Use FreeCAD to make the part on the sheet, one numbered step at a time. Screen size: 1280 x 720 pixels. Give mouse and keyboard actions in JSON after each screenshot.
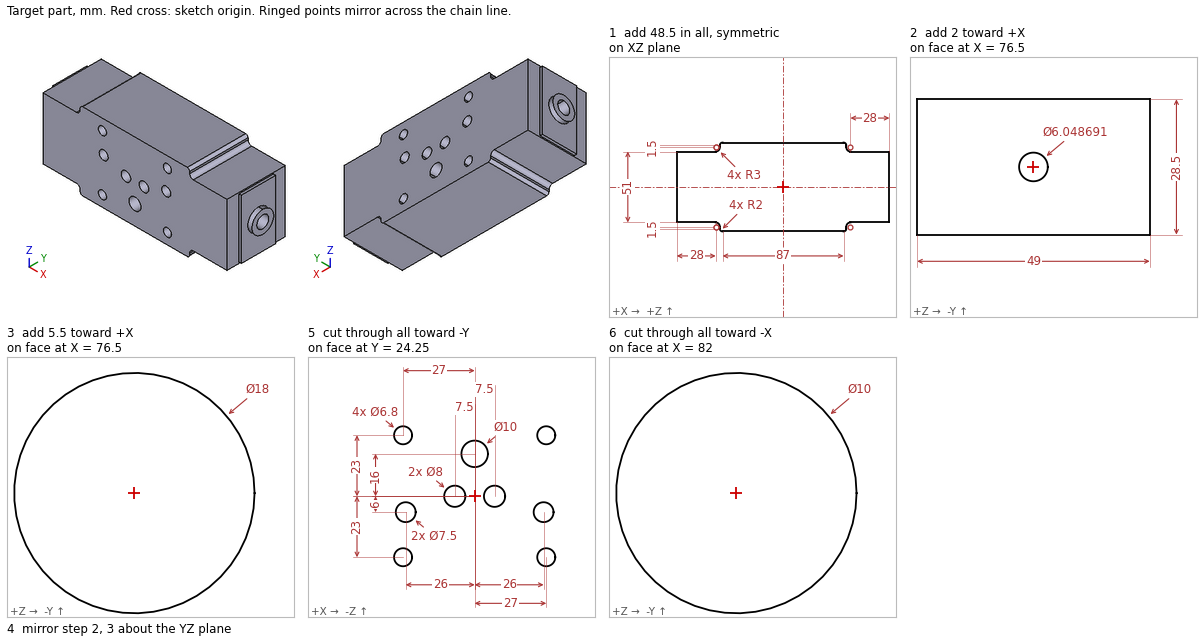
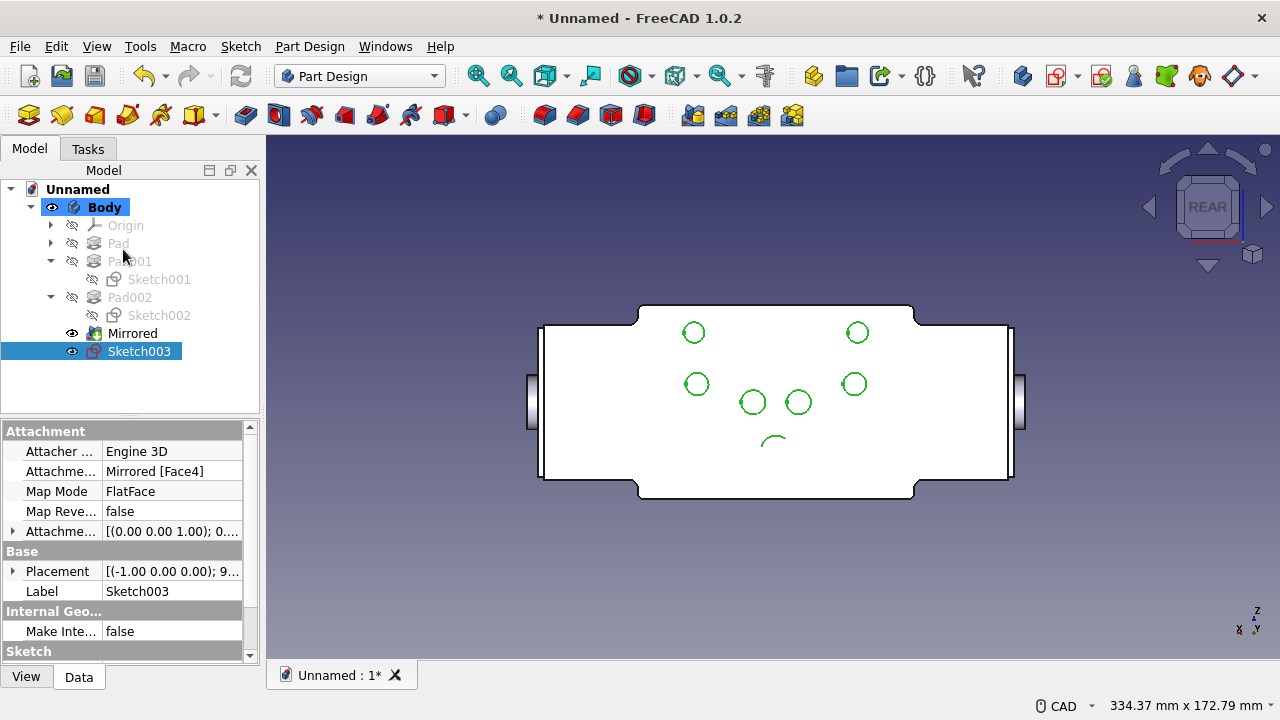
{"action": "left_click", "coordinate": [246, 116]}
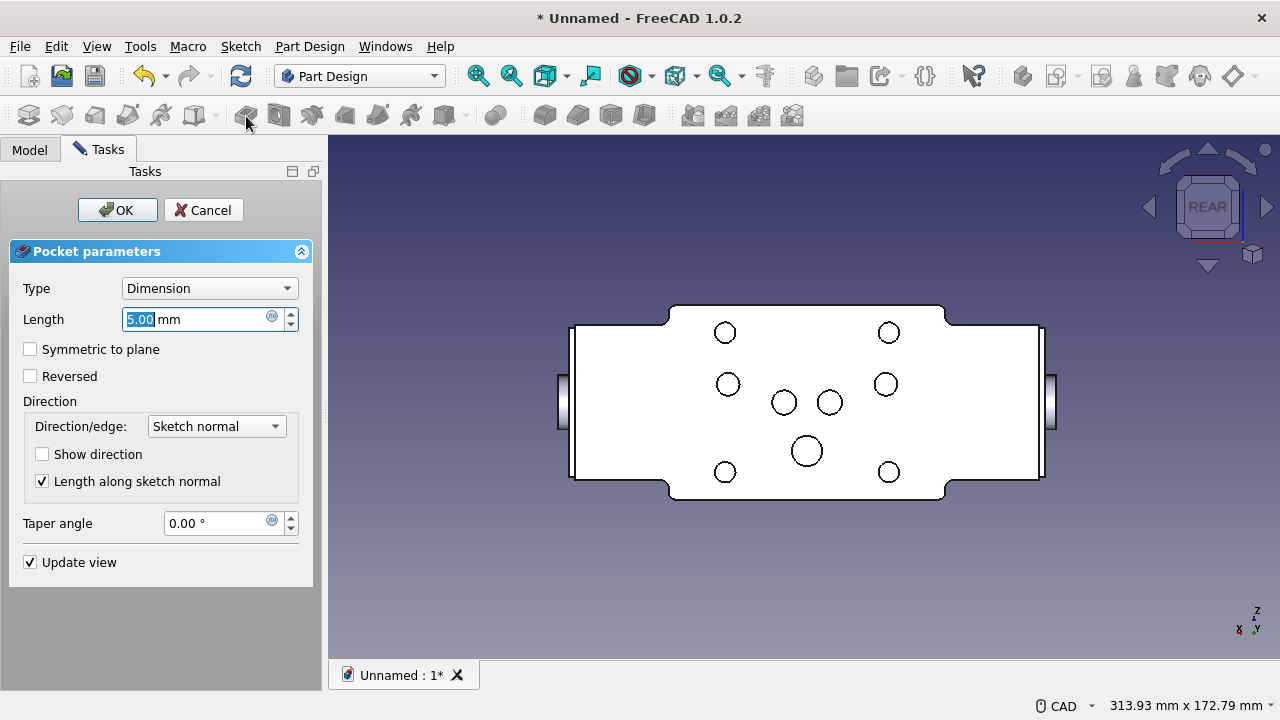
{"action": "left_click", "coordinate": [210, 288]}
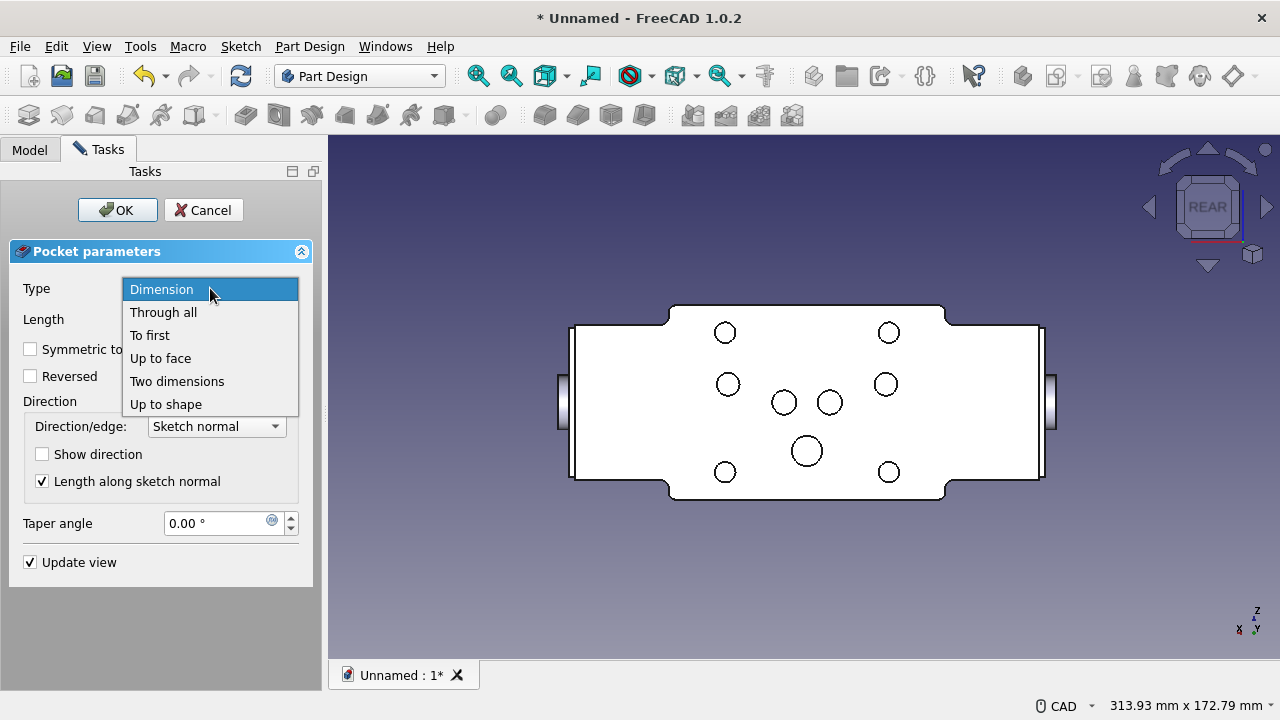
{"action": "left_click", "coordinate": [208, 312]}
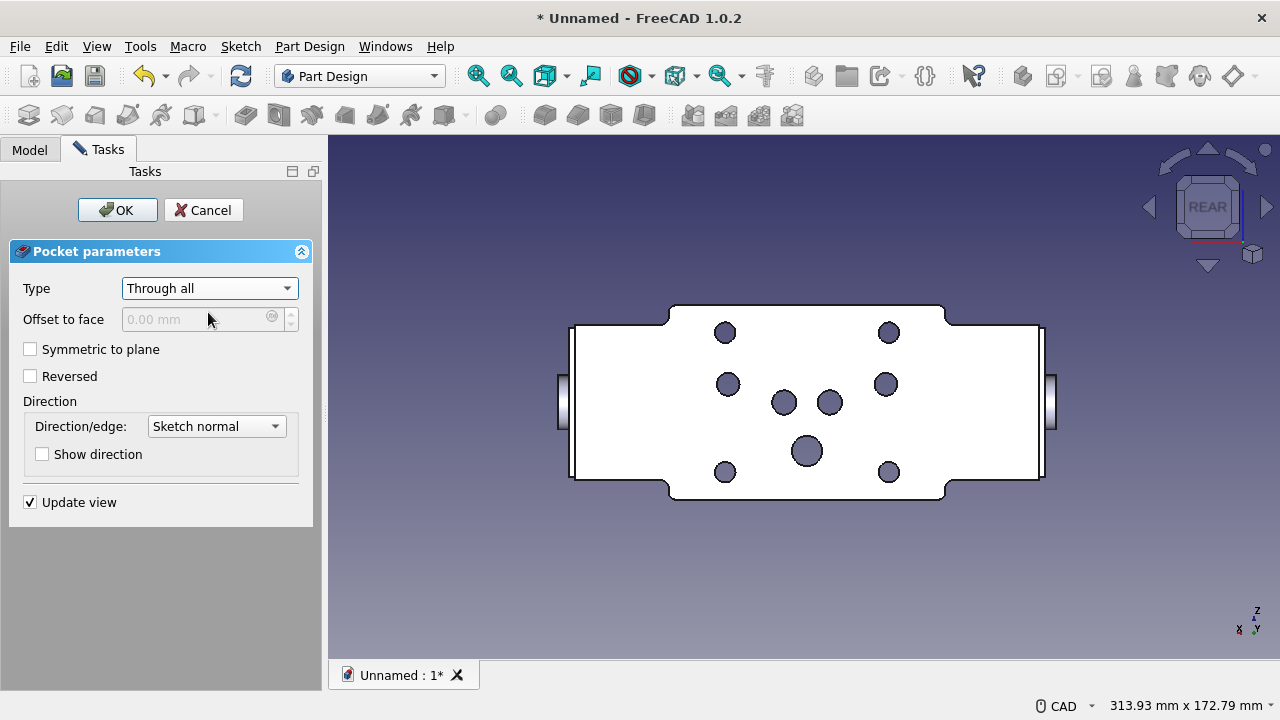
{"action": "left_click", "coordinate": [118, 210]}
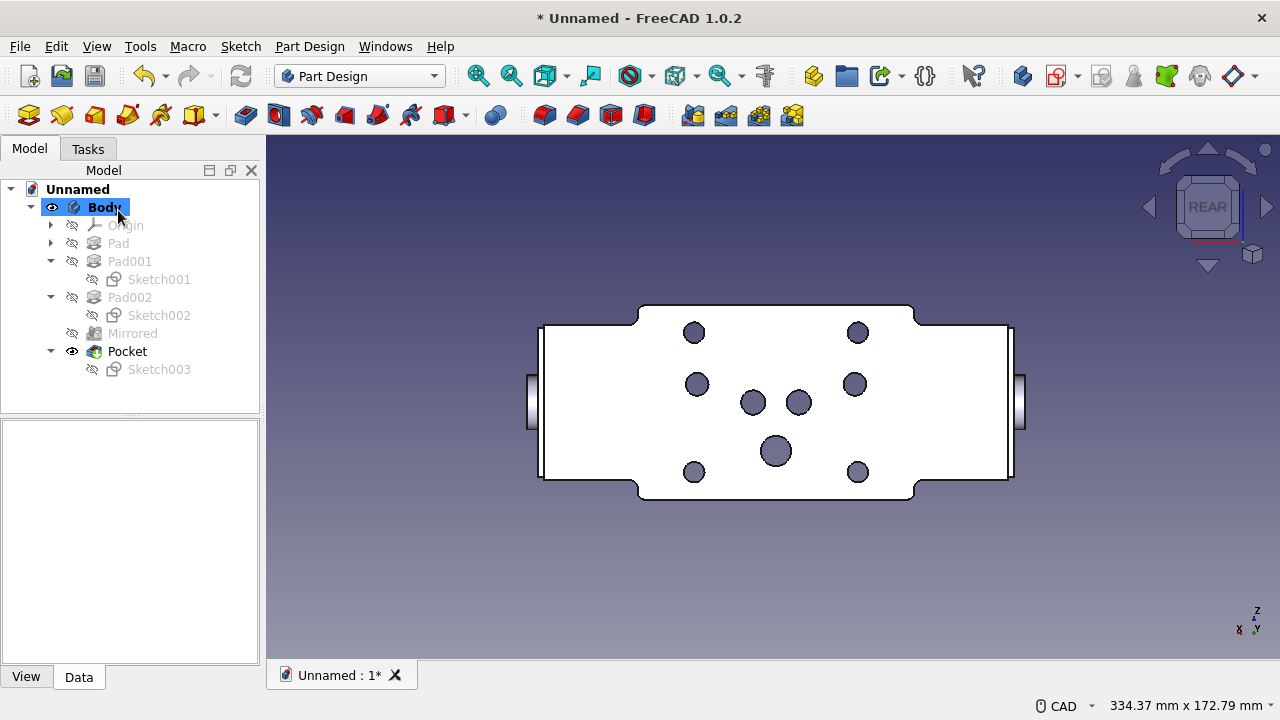
{"action": "key", "text": "0"}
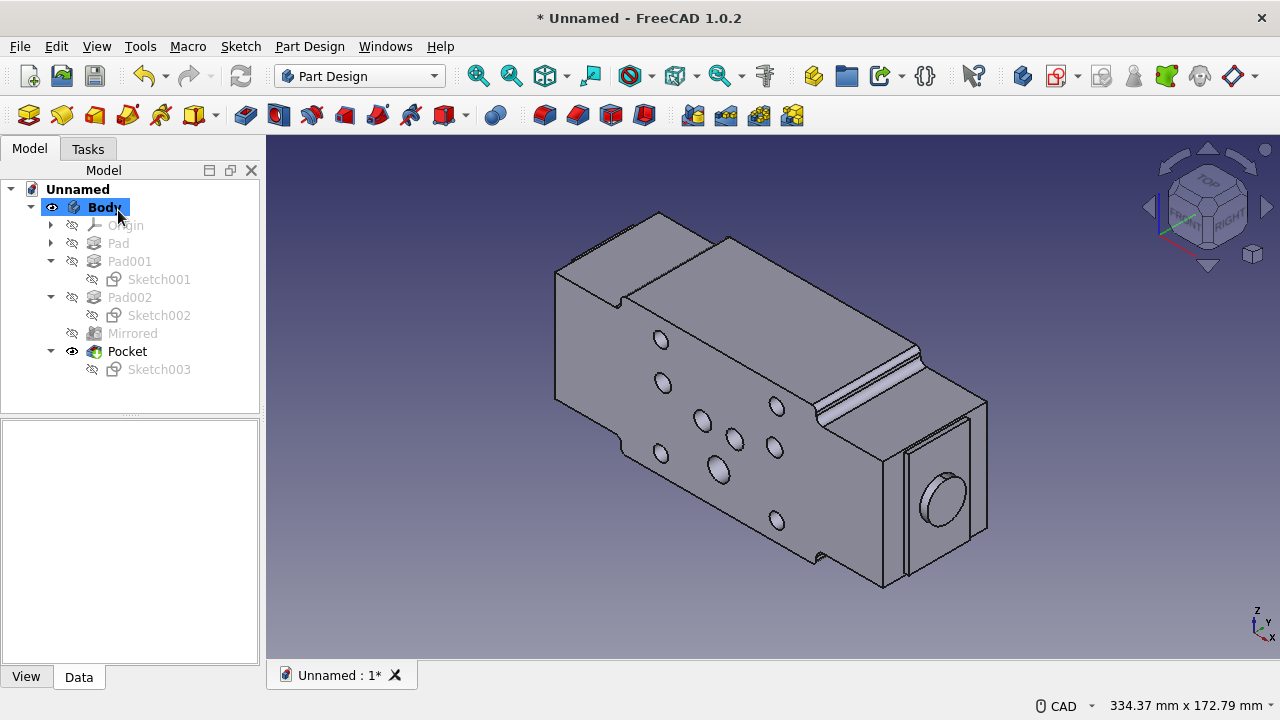
{"action": "left_click", "coordinate": [947, 501]}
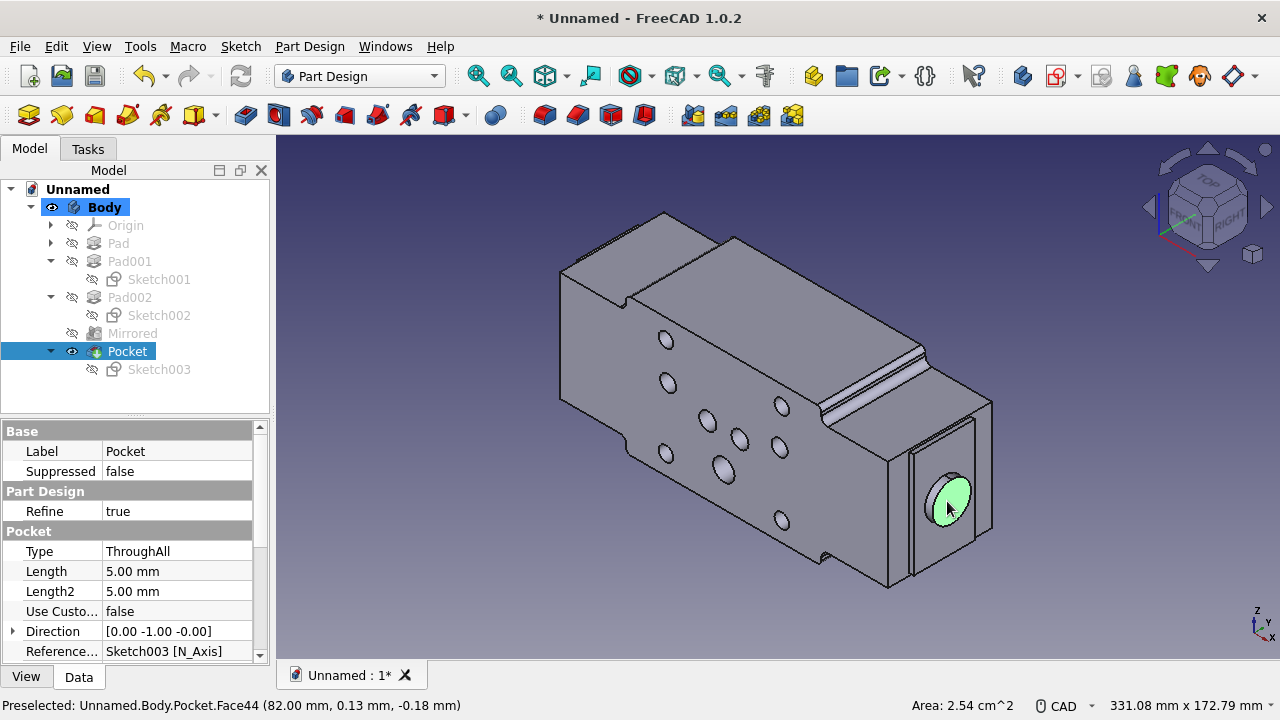
{"action": "left_click", "coordinate": [1056, 76]}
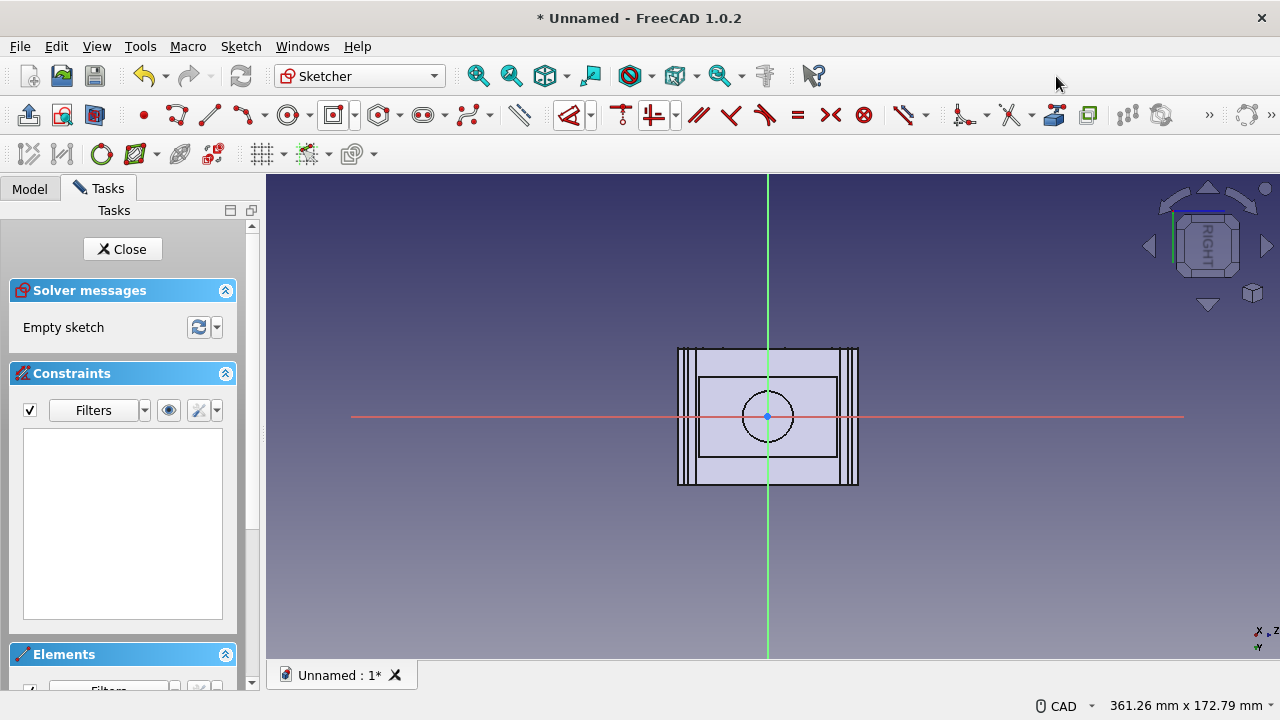
{"action": "scroll", "coordinate": [774, 417], "scroll_direction": "up", "scroll_amount": 12}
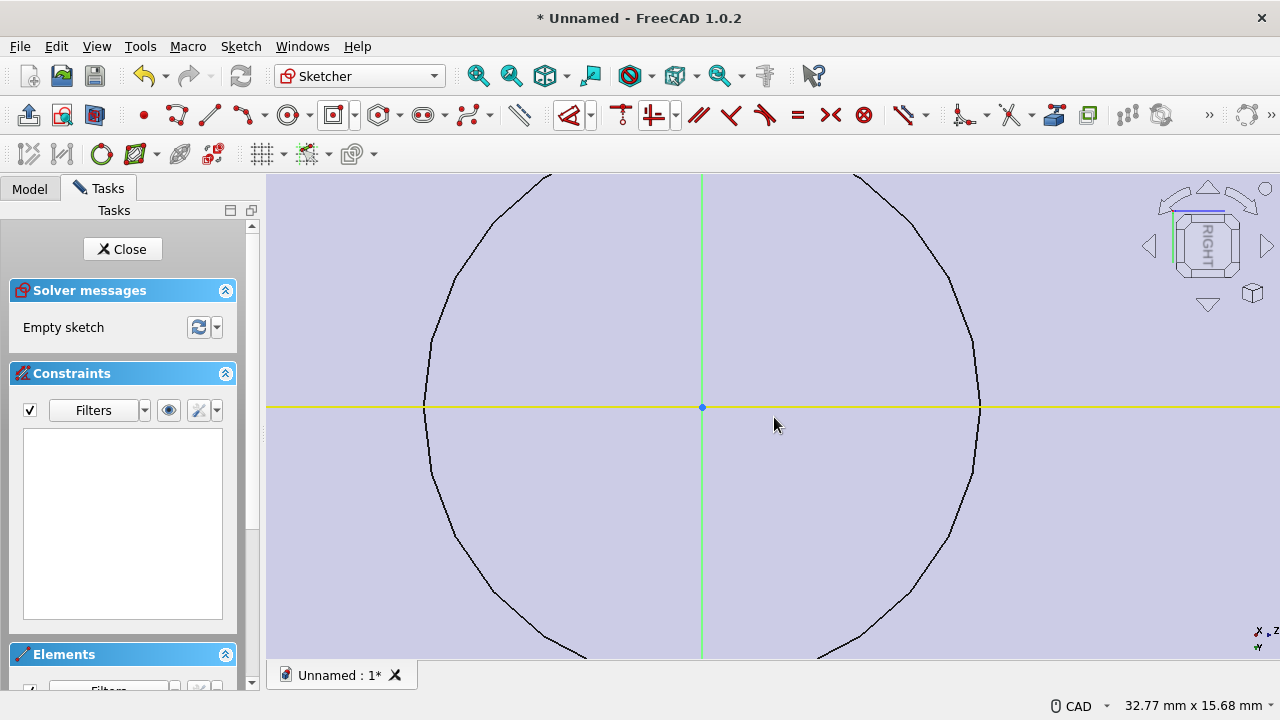
{"action": "left_click", "coordinate": [288, 116]}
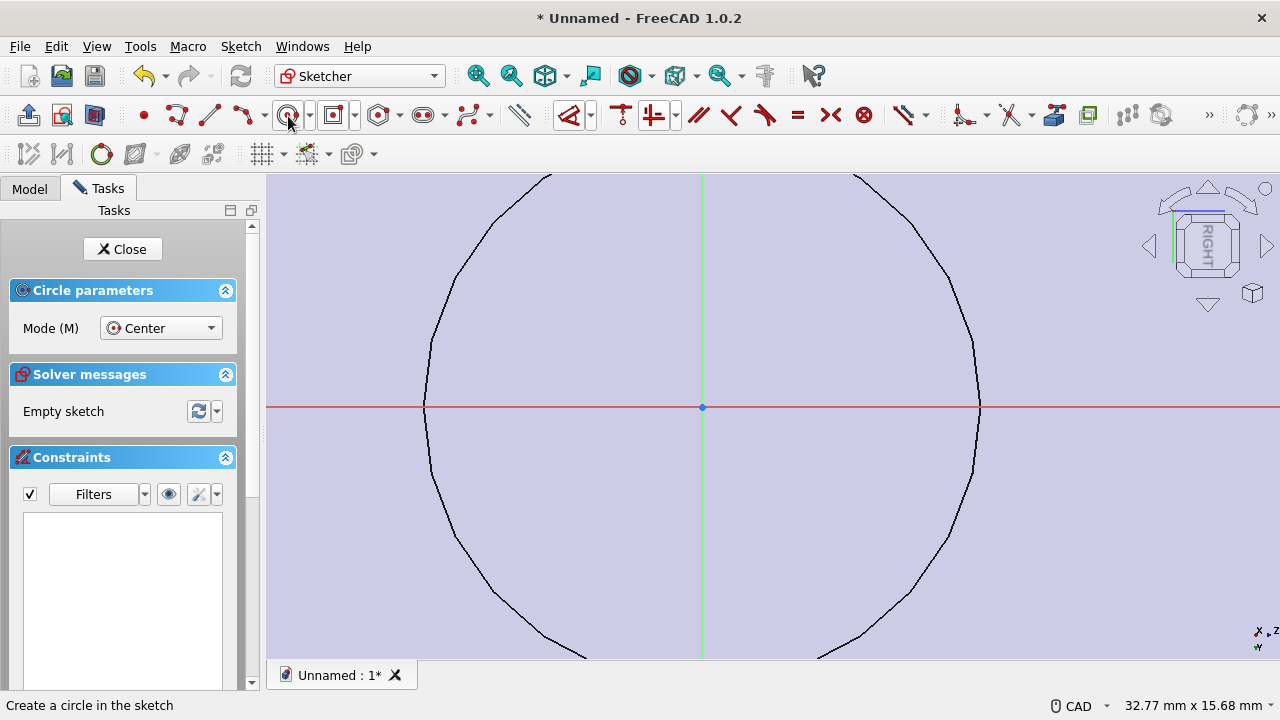
{"action": "left_click", "coordinate": [702, 407]}
{"action": "left_click", "coordinate": [811, 298]}
{"action": "key", "text": "Escape"}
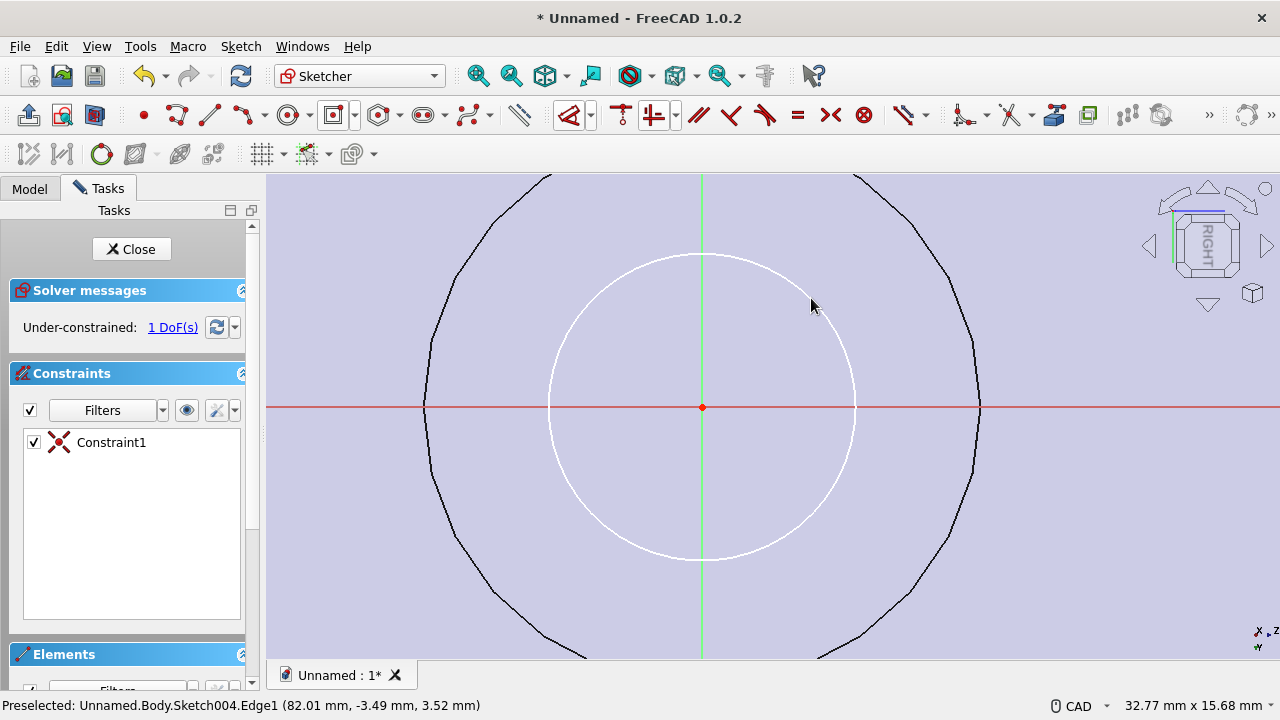
{"action": "left_click", "coordinate": [810, 298]}